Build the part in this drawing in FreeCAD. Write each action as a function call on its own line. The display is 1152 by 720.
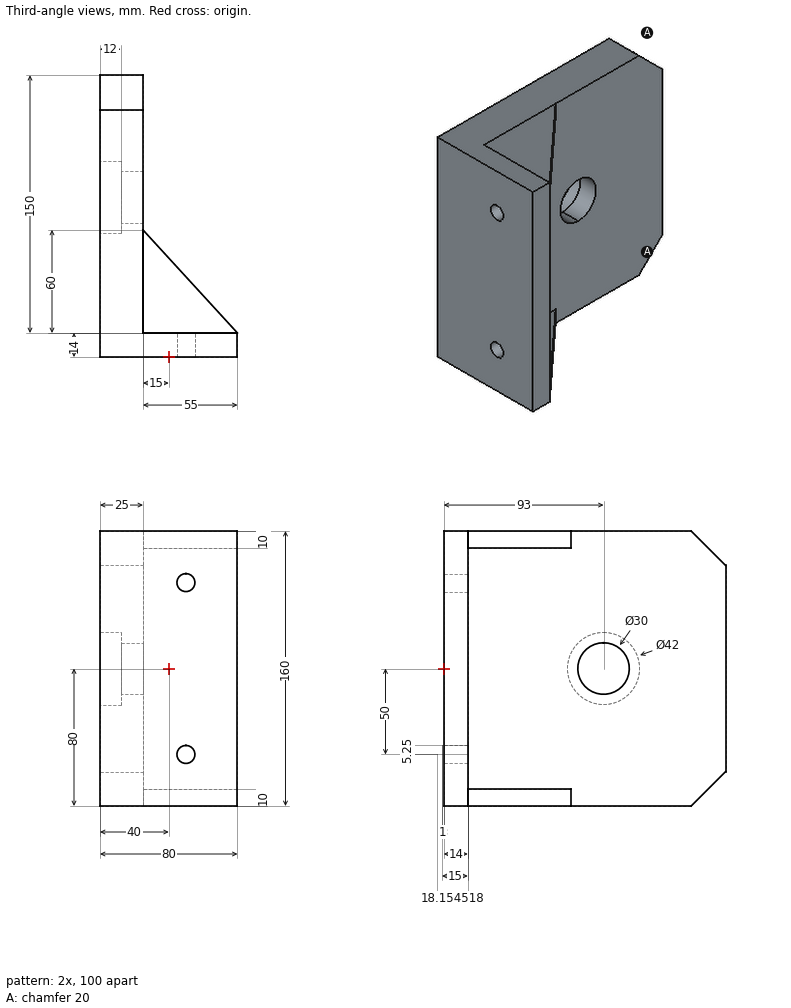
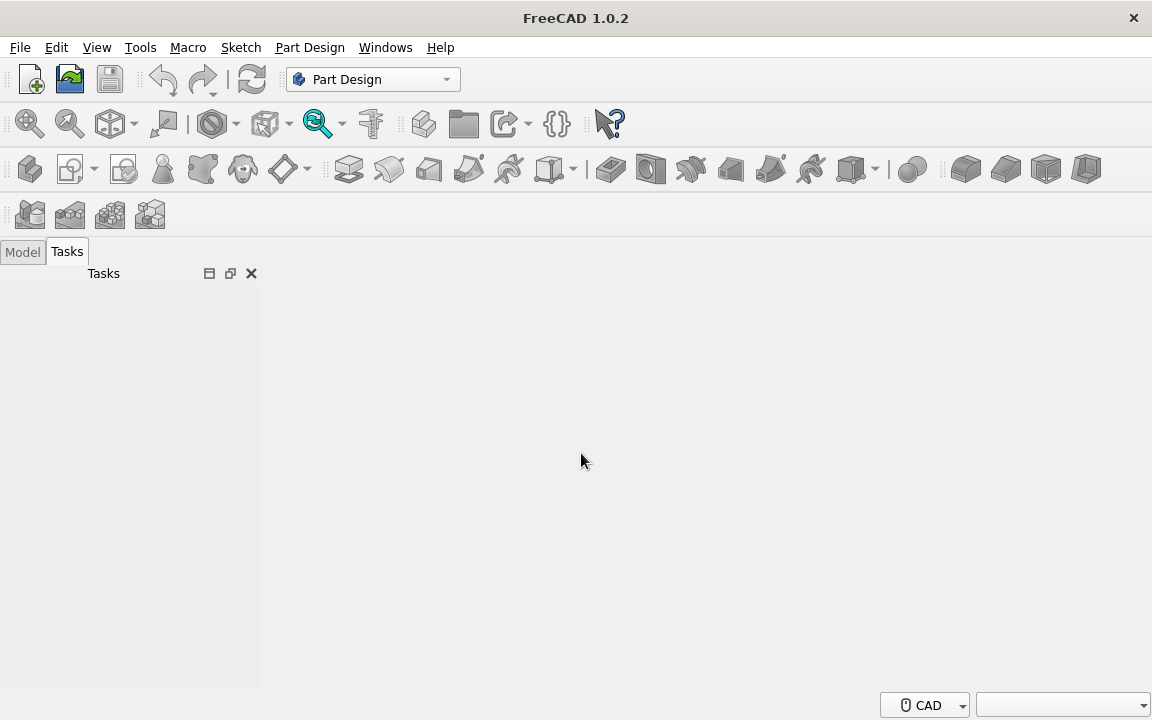
click(30, 80)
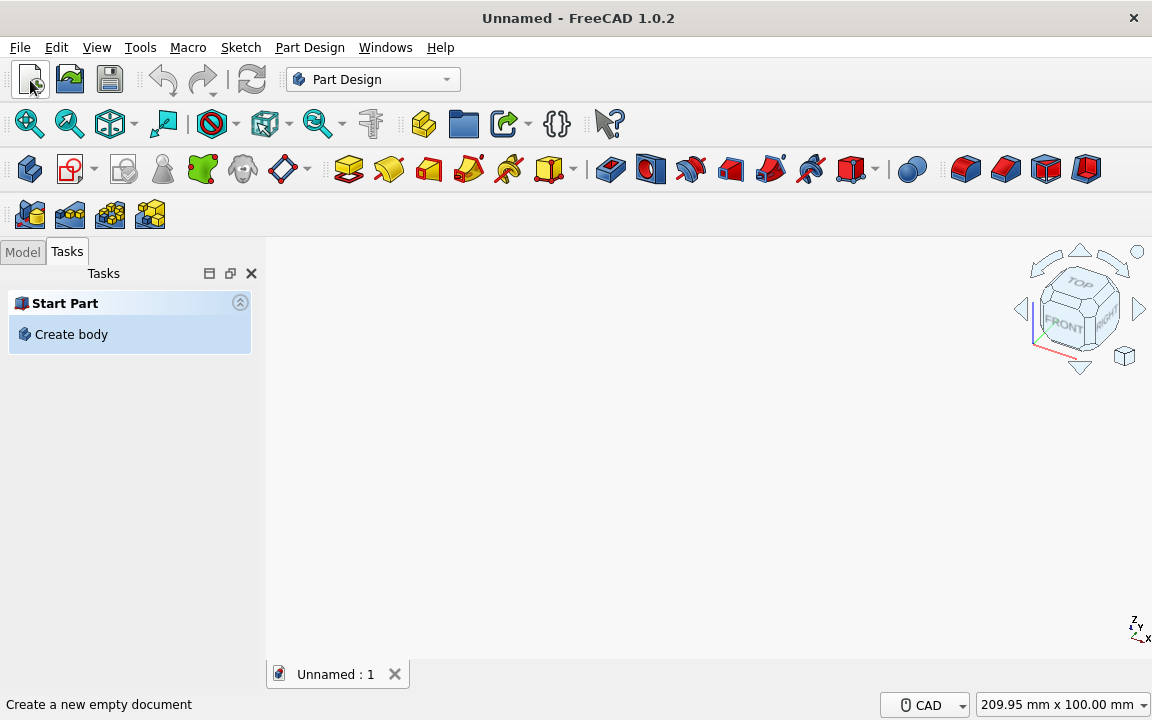
click(70, 170)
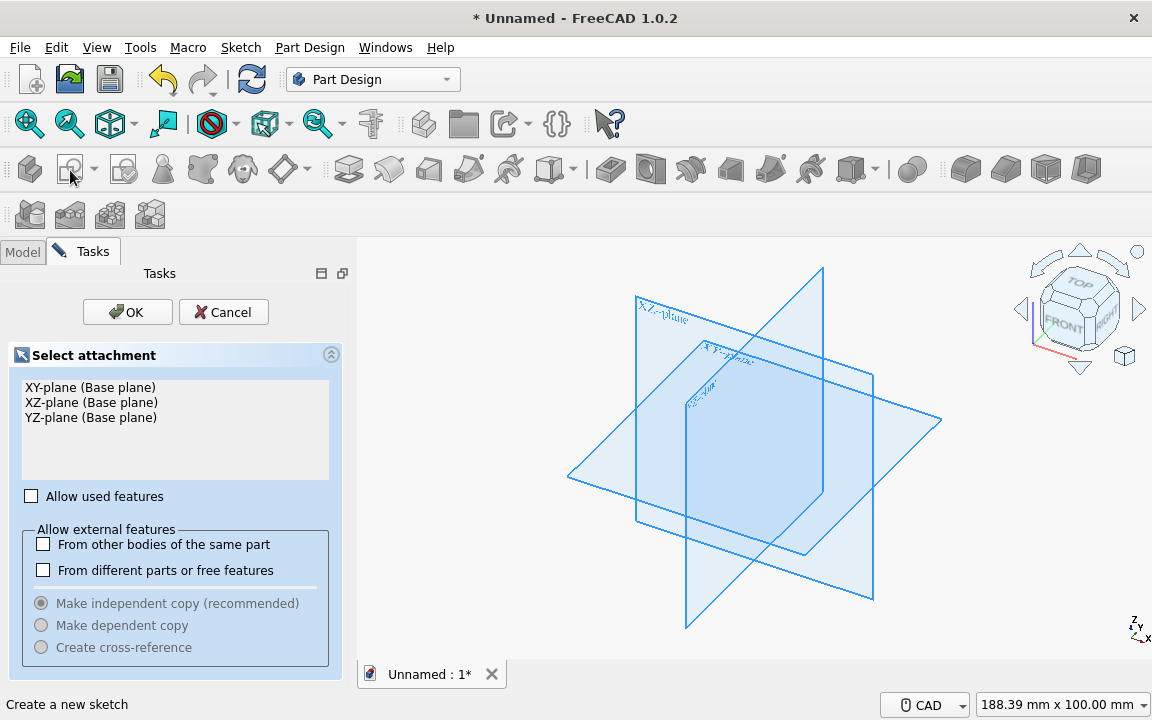
click(82, 402)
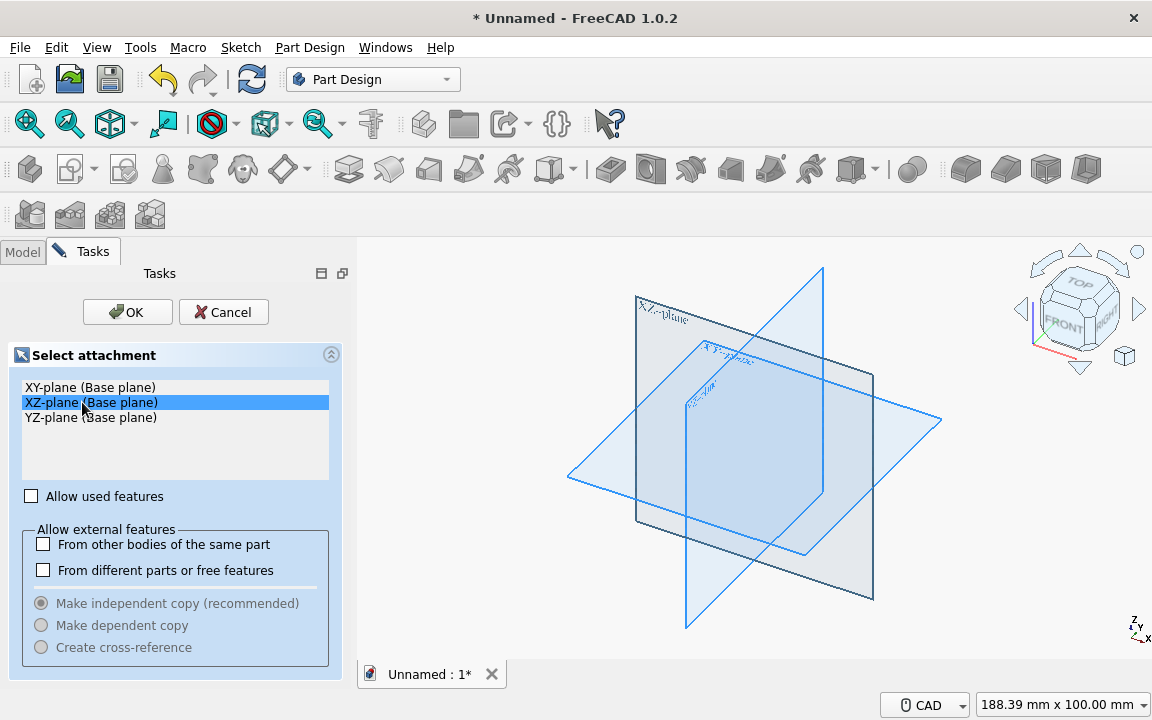
click(128, 312)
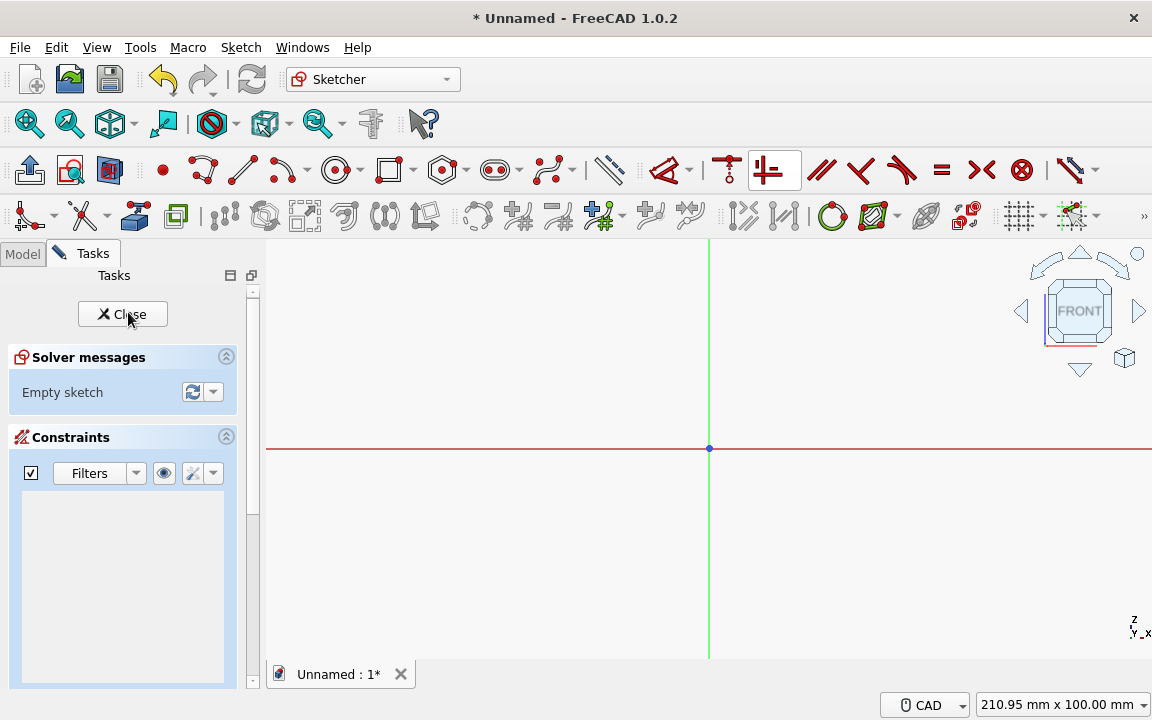
scroll(601, 449, down, 5)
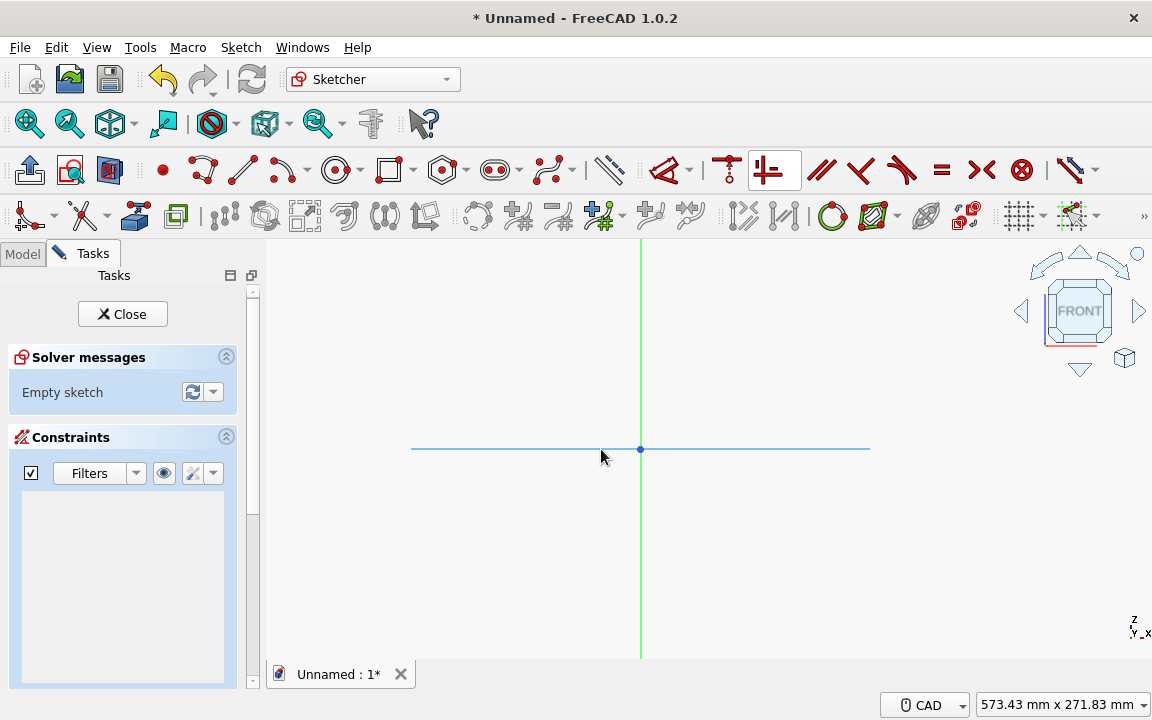
click(416, 170)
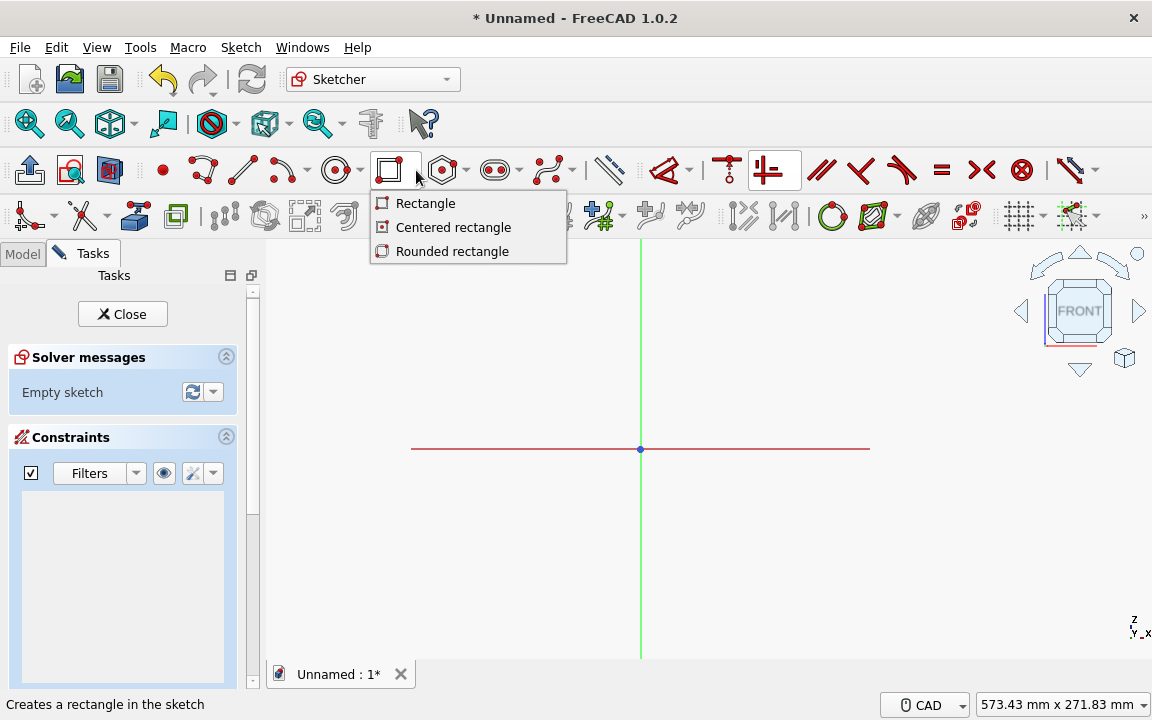
click(468, 227)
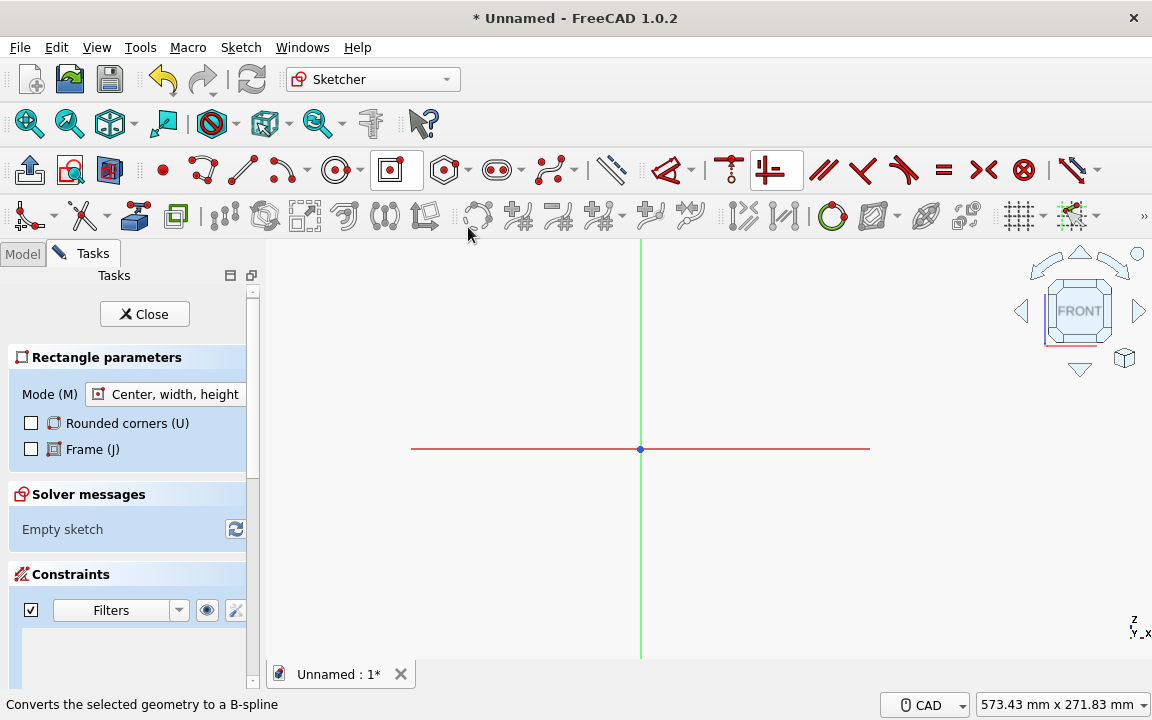
click(641, 449)
move(703, 326)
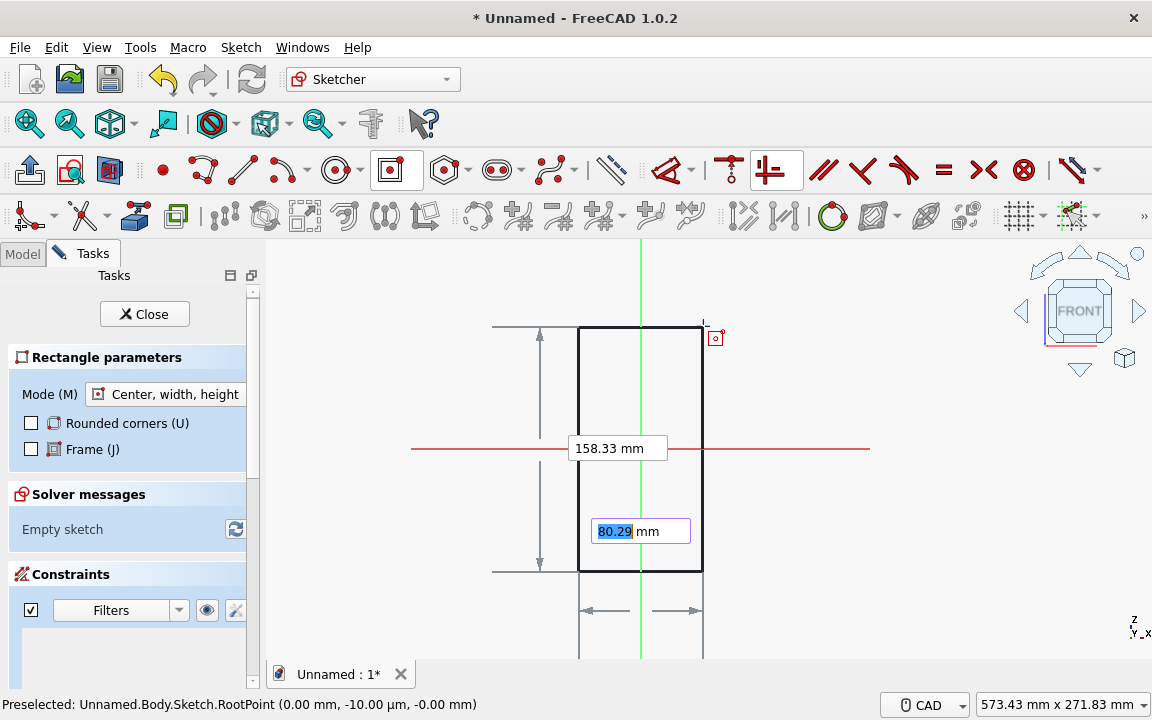
text(80)
key(Tab)
text(160)
key(Return)
key(Escape)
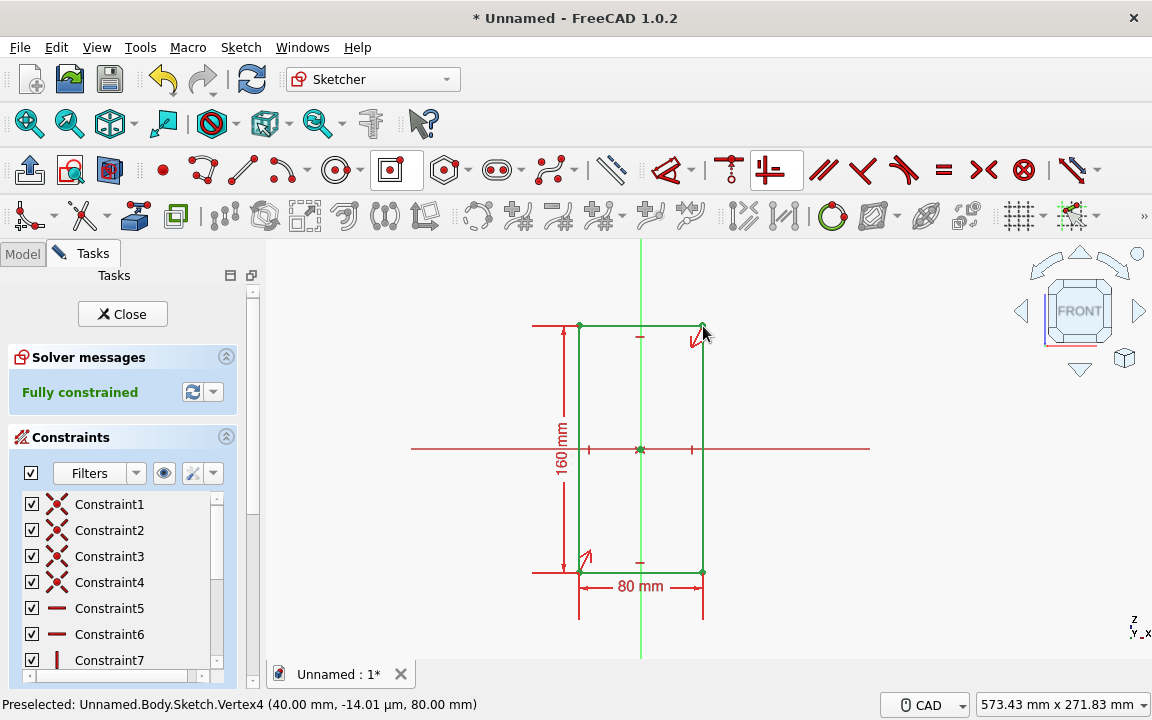
click(123, 314)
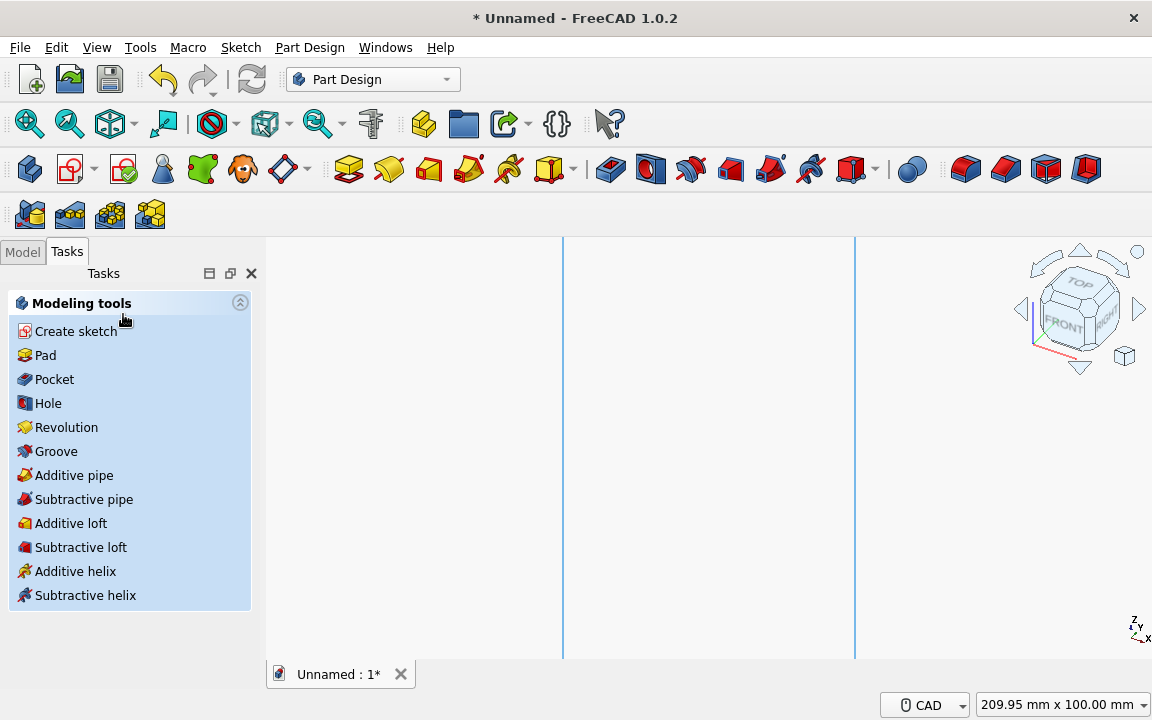
click(350, 170)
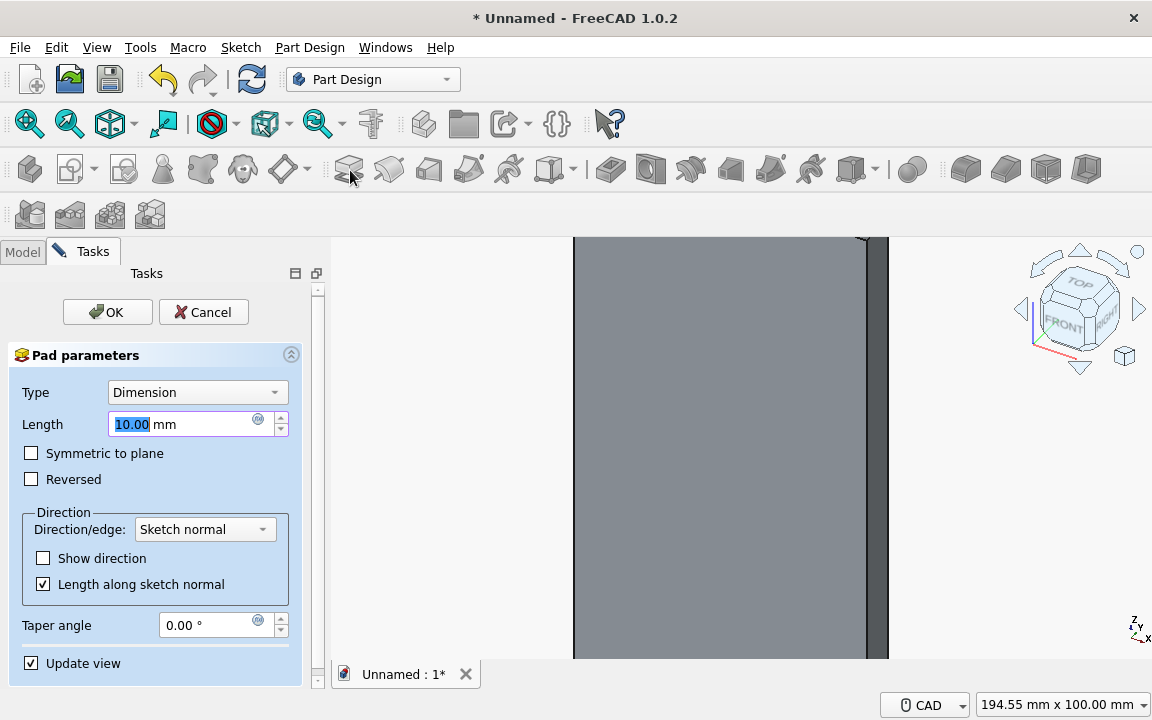
text(14)
key(Tab)